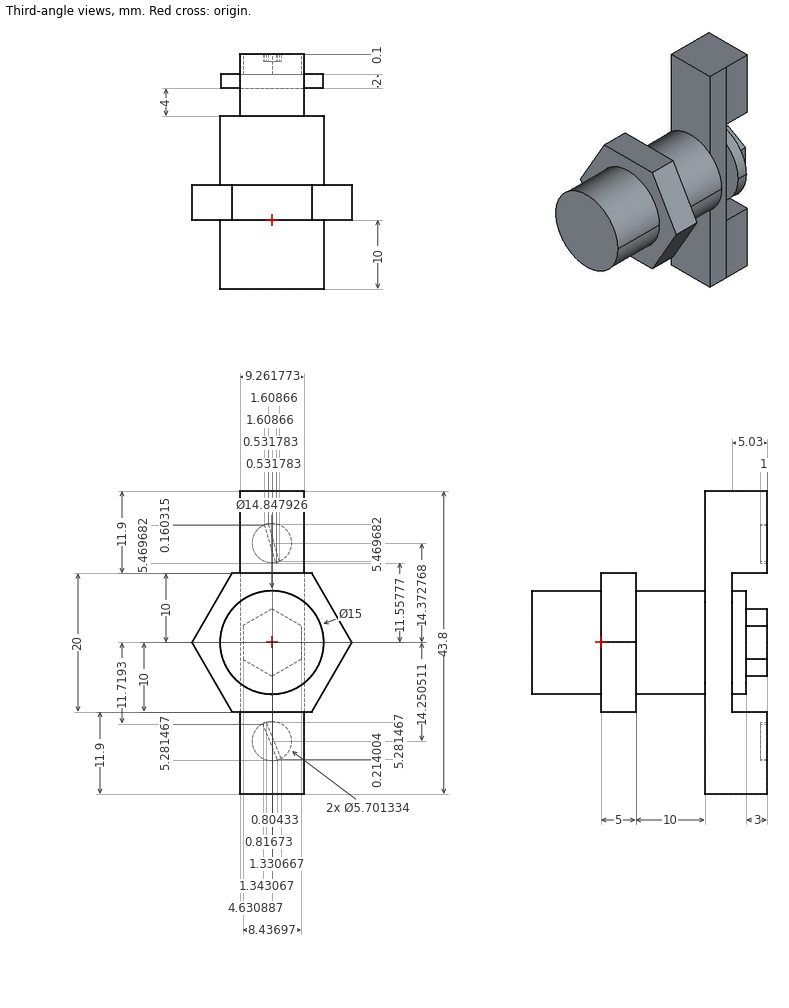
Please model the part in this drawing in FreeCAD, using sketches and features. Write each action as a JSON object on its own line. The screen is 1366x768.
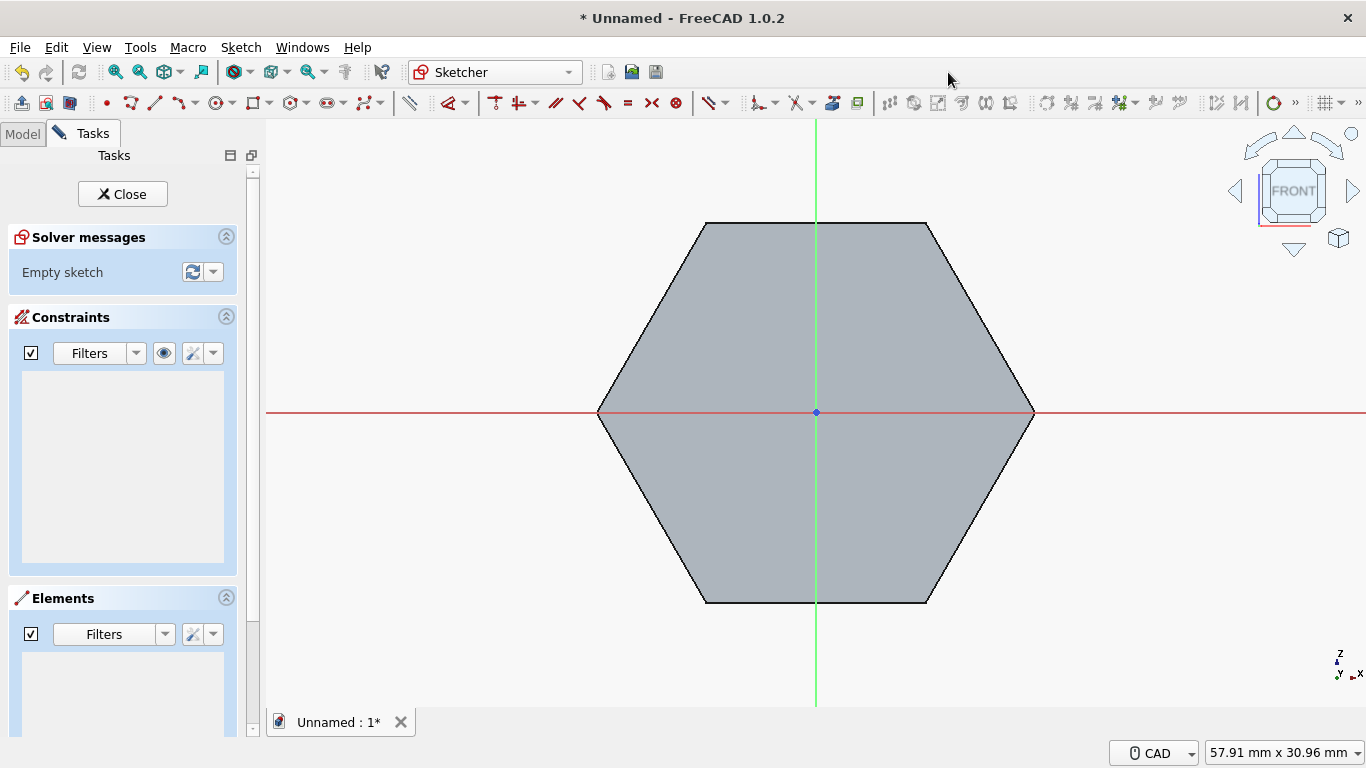
{"action": "left_click", "coordinate": [216, 104]}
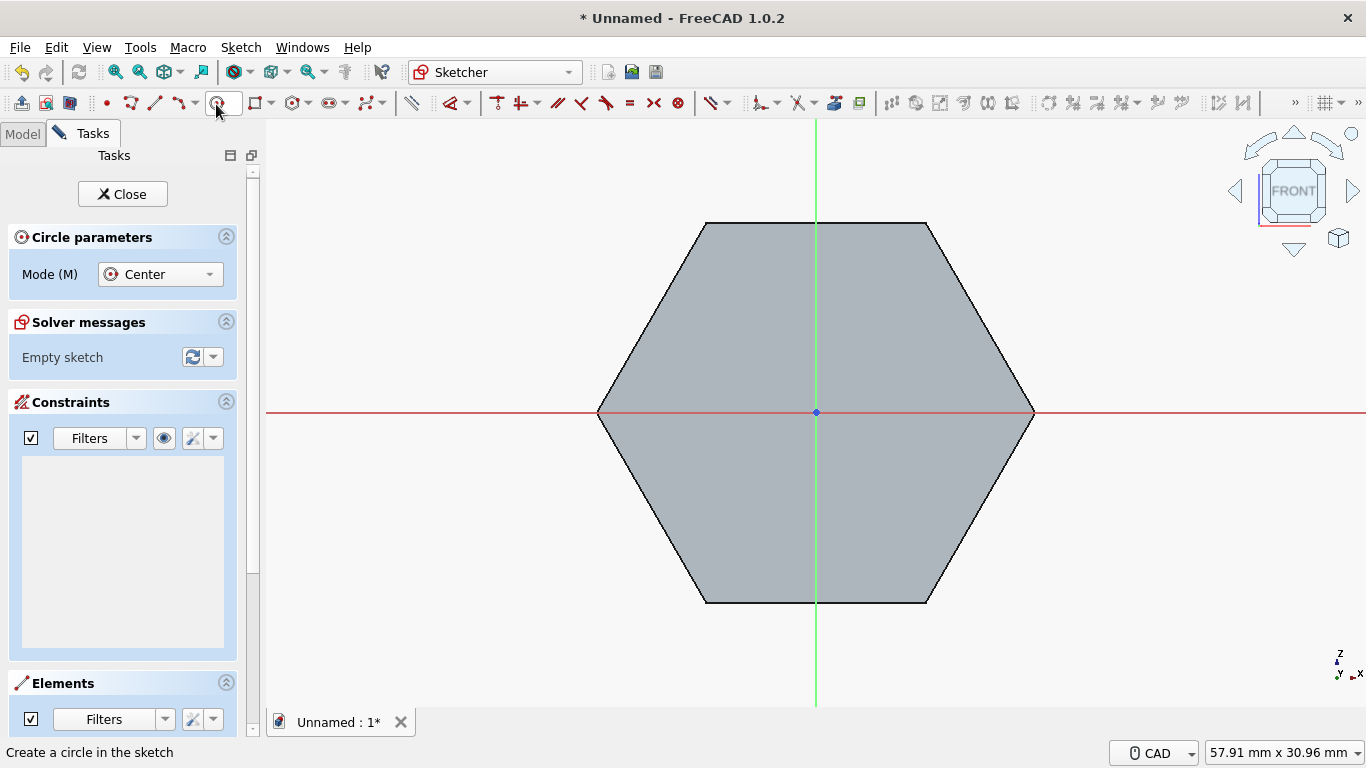
{"action": "left_click", "coordinate": [816, 413]}
{"action": "left_click", "coordinate": [917, 312]}
{"action": "key", "text": "Escape"}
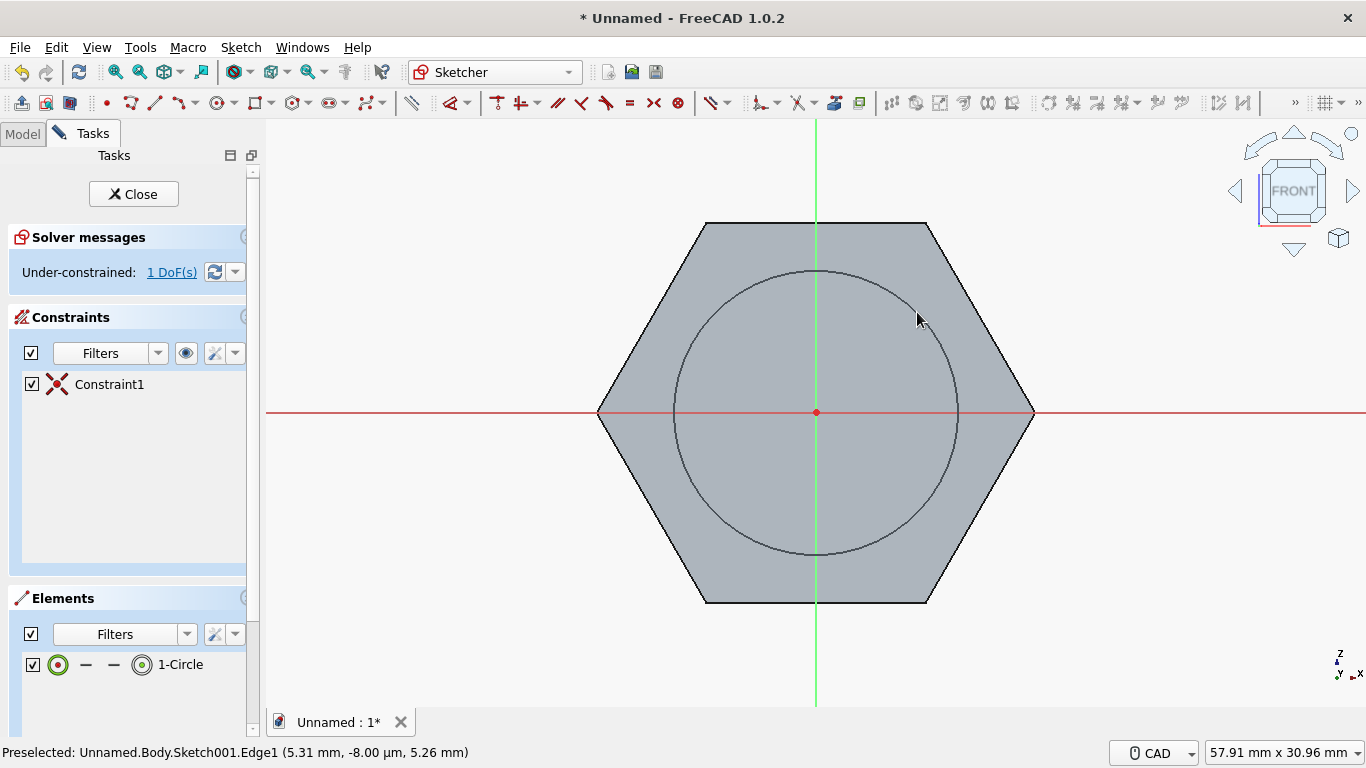
{"action": "left_click", "coordinate": [450, 104]}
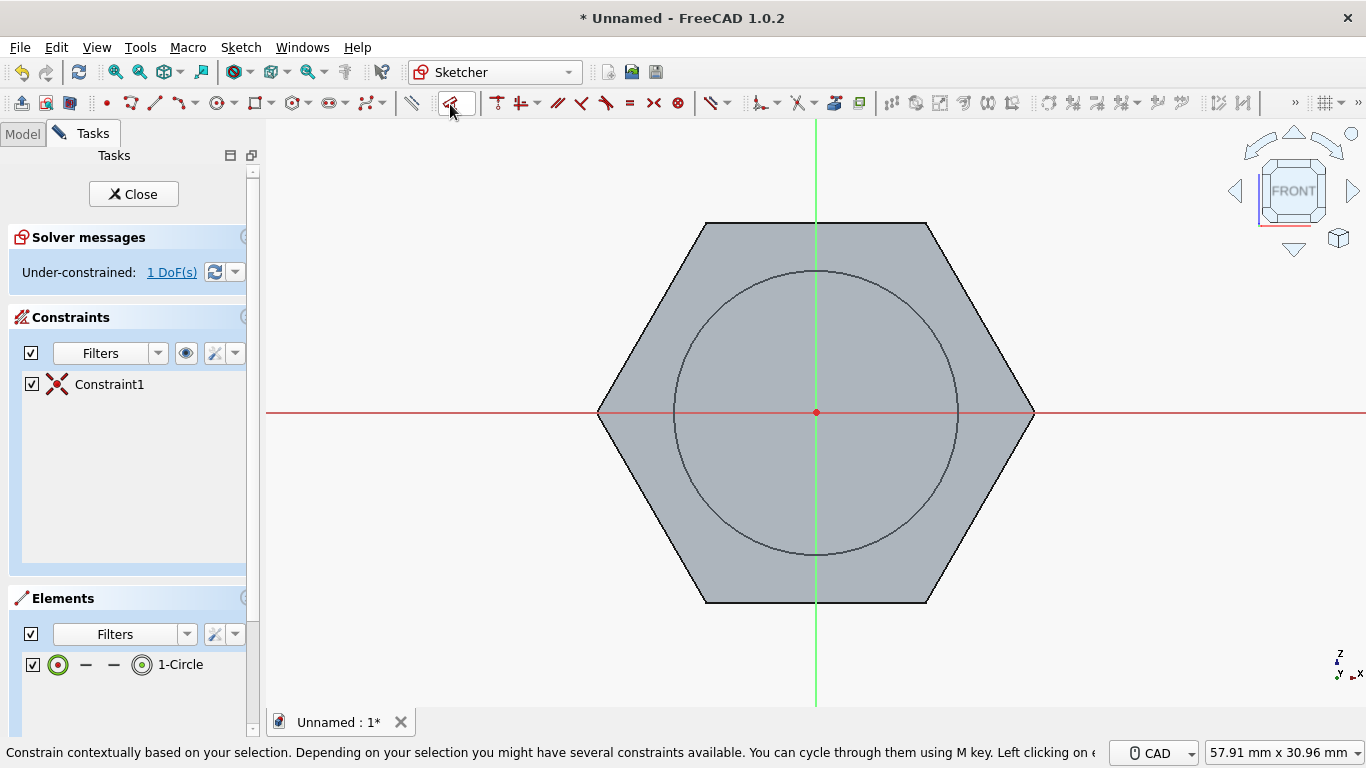
{"action": "left_click", "coordinate": [916, 312]}
{"action": "left_click", "coordinate": [939, 289]}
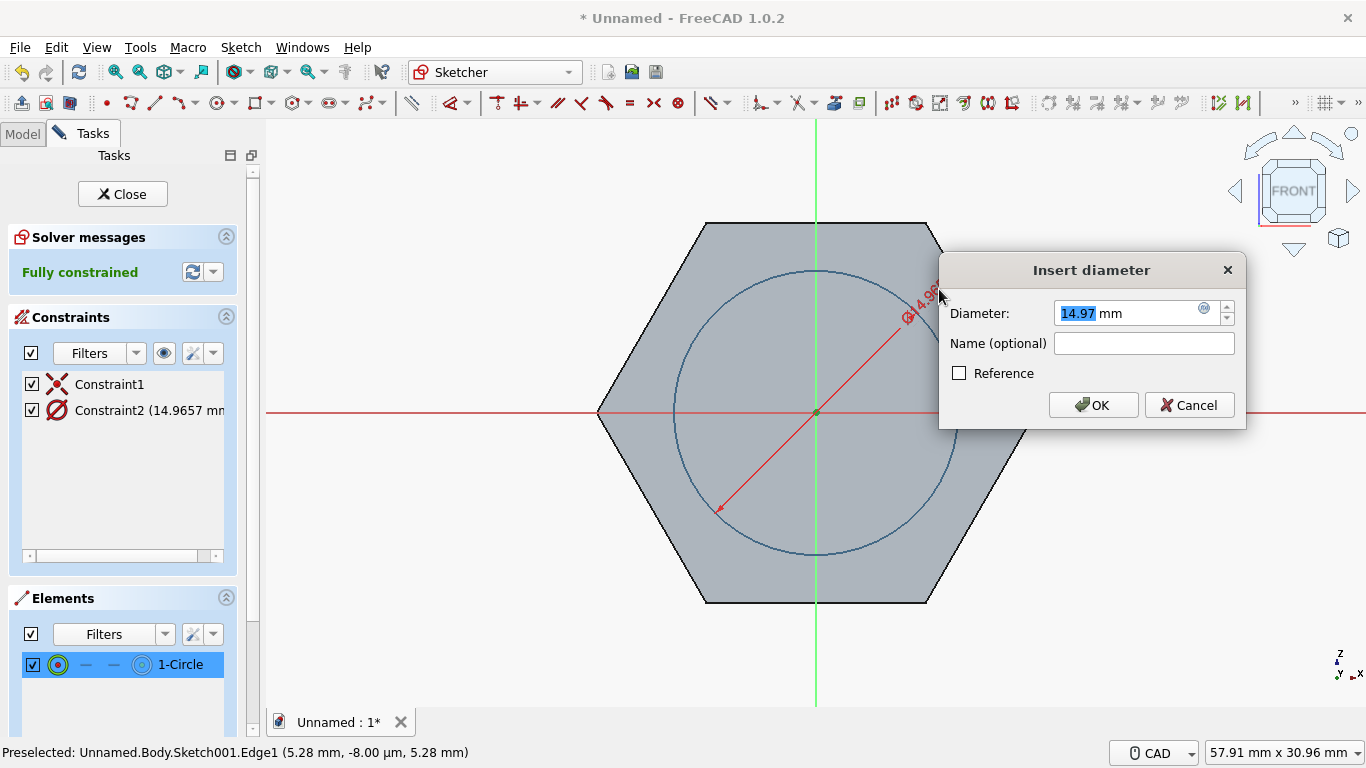
{"action": "type", "text": "15"}
{"action": "key", "text": "Return"}
{"action": "key", "text": "Escape"}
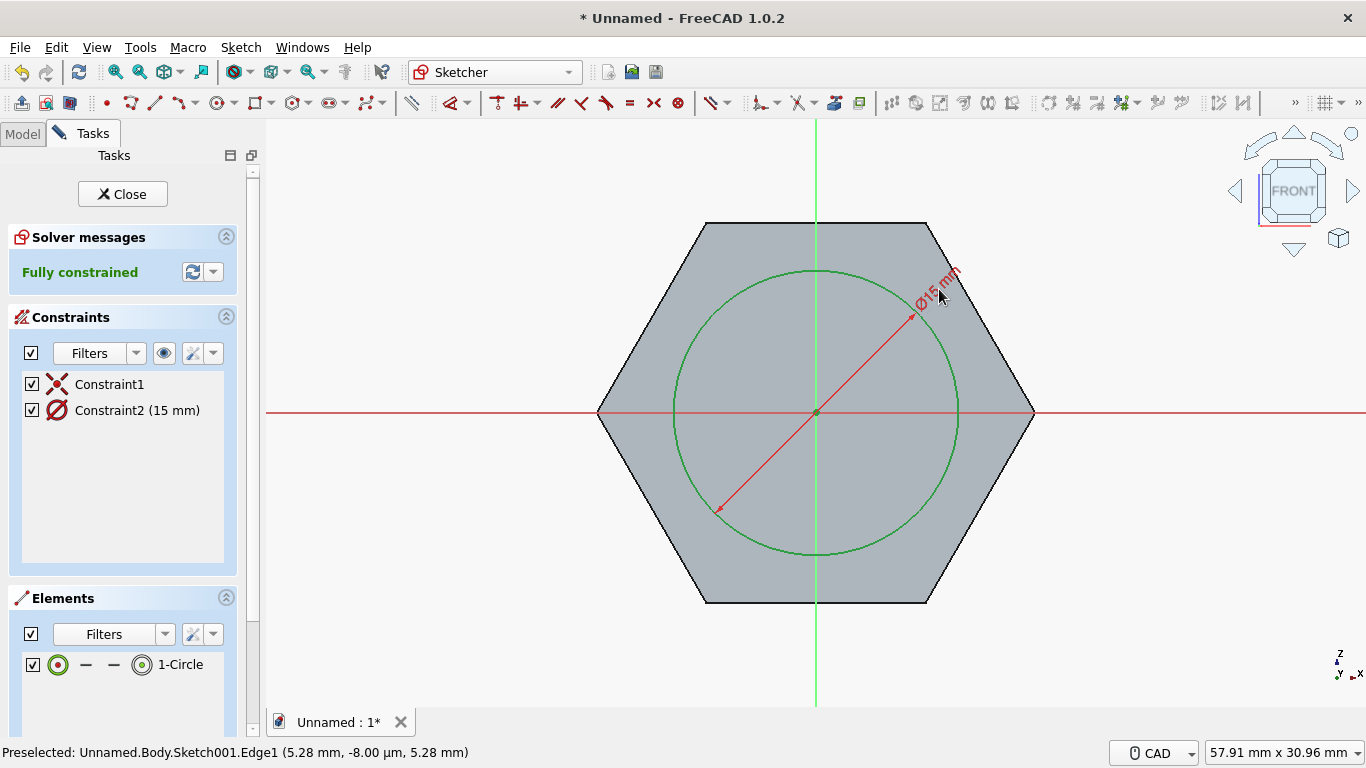
{"action": "left_click", "coordinate": [123, 194]}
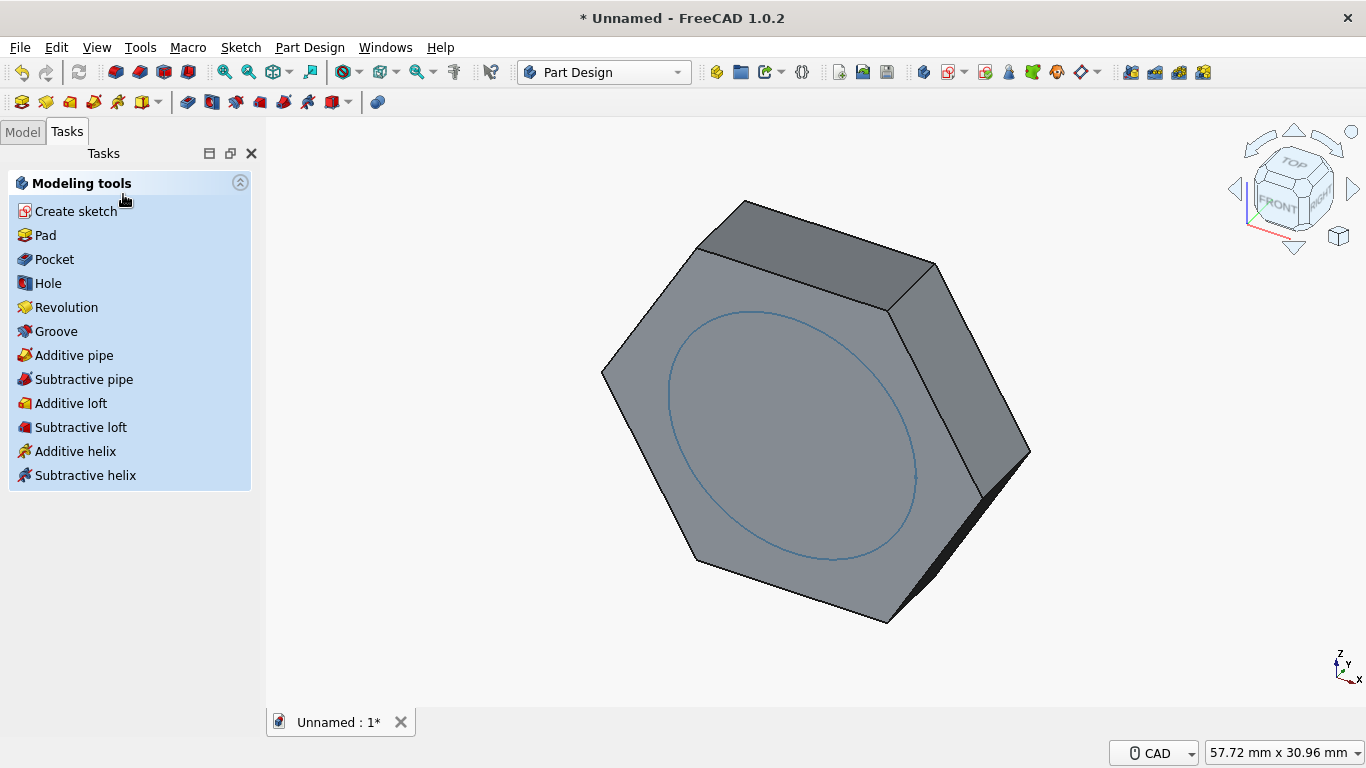
{"action": "left_click", "coordinate": [22, 102]}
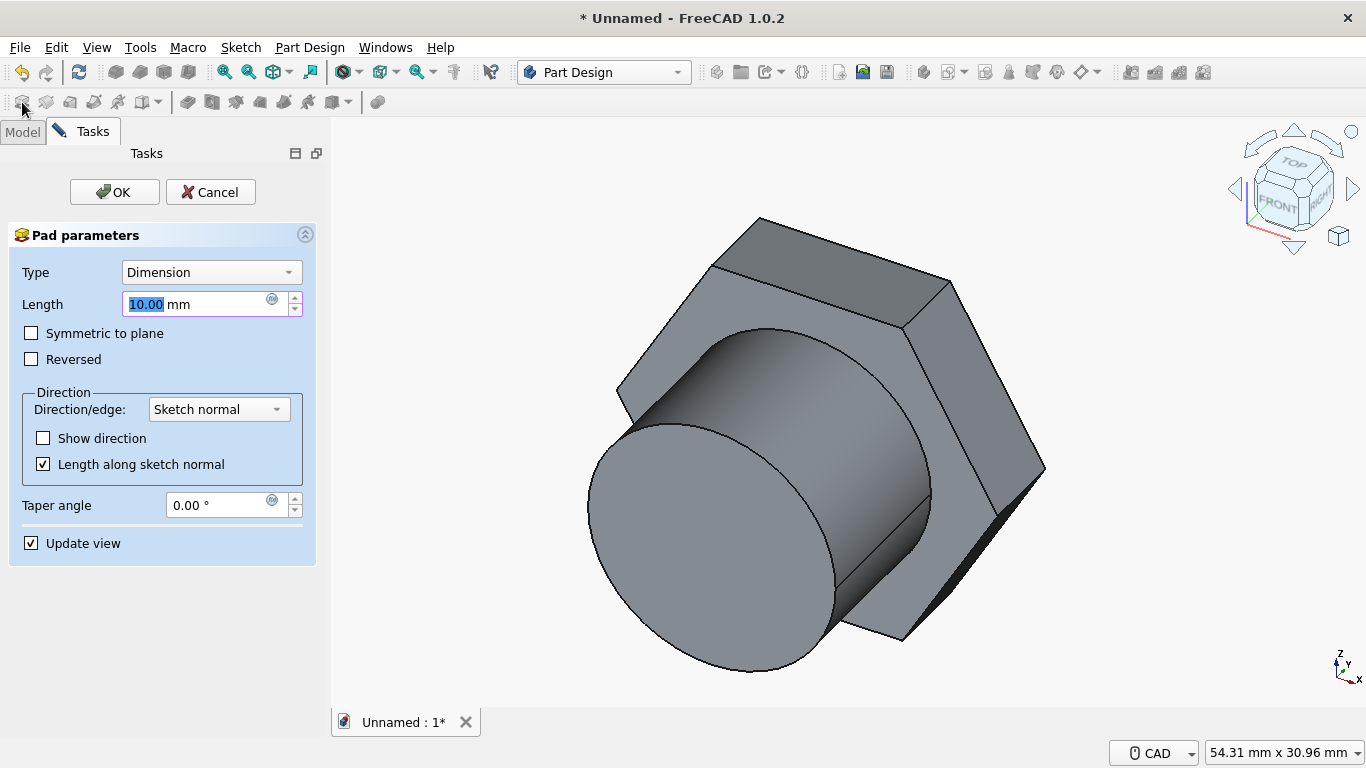
{"action": "type", "text": "10"}
{"action": "key", "text": "Tab"}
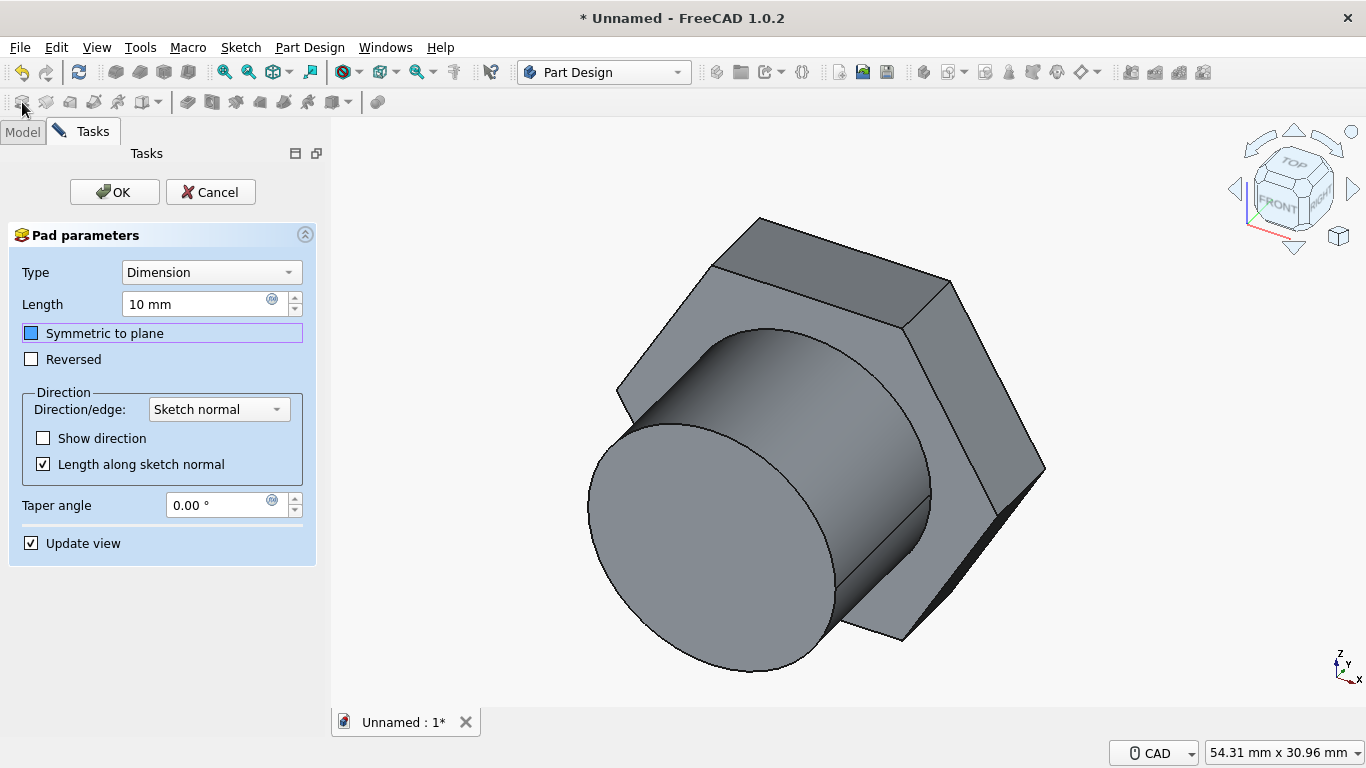
{"action": "left_click", "coordinate": [115, 192]}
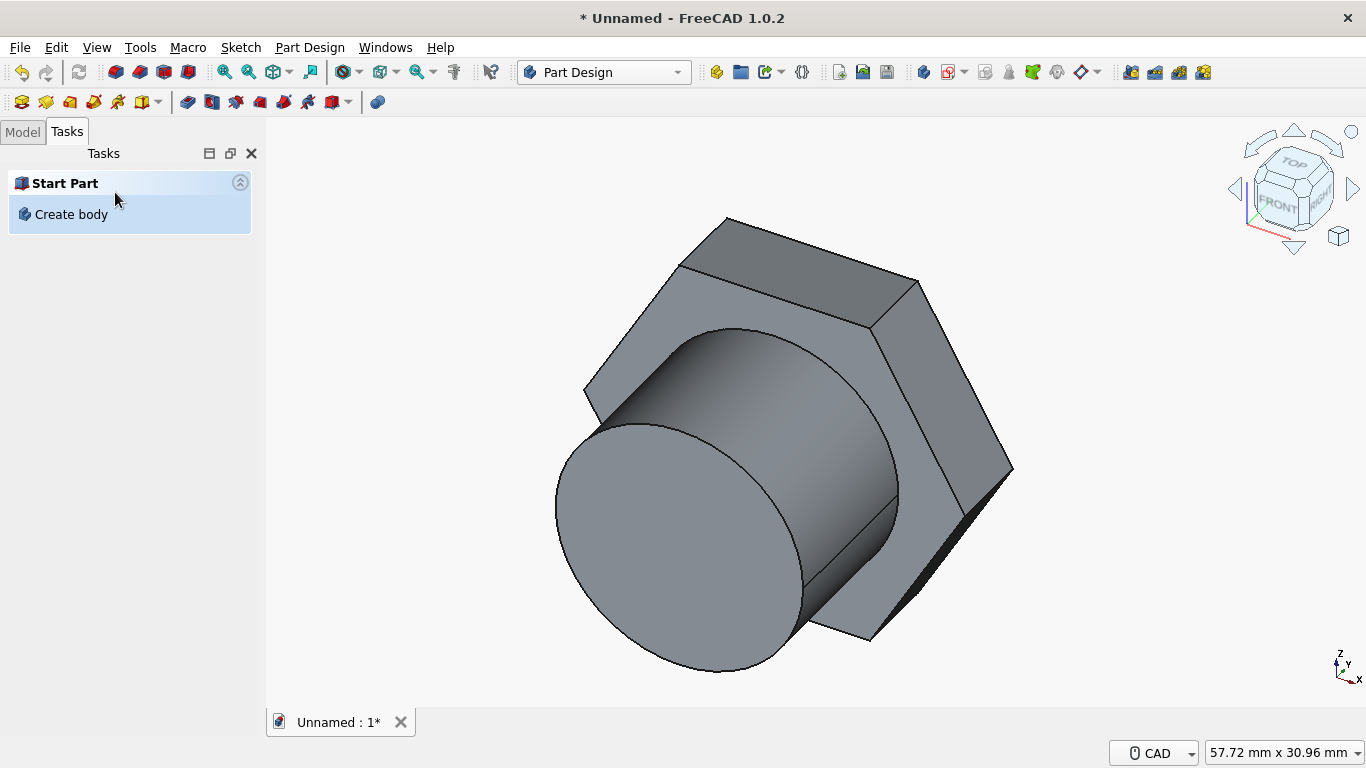
{"action": "left_click", "coordinate": [226, 72]}